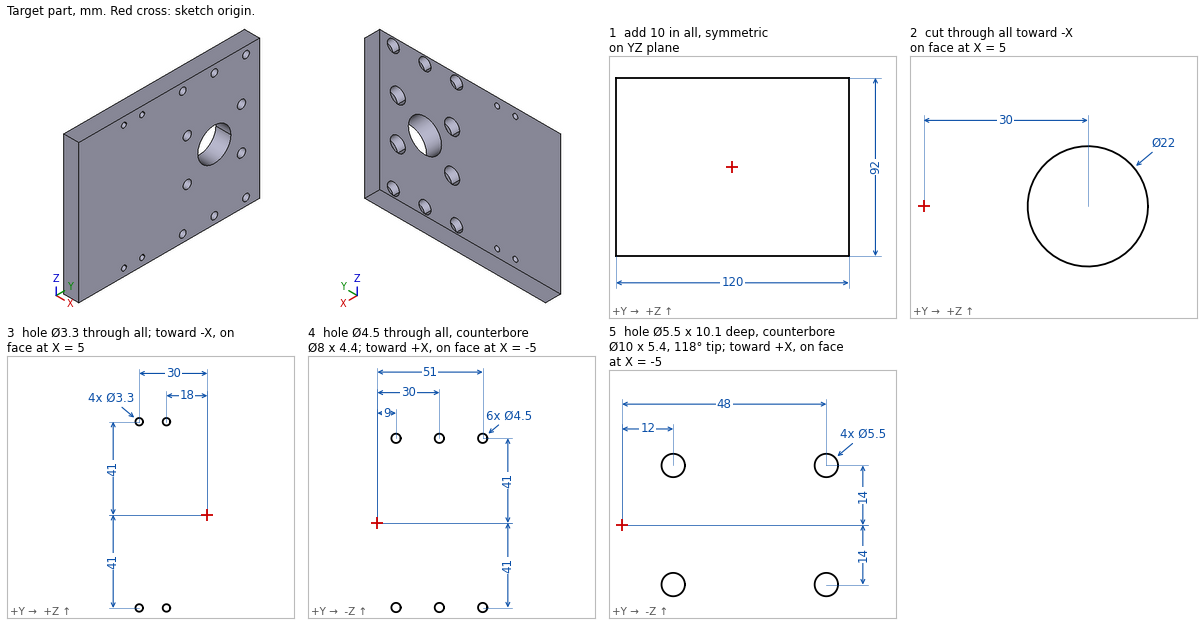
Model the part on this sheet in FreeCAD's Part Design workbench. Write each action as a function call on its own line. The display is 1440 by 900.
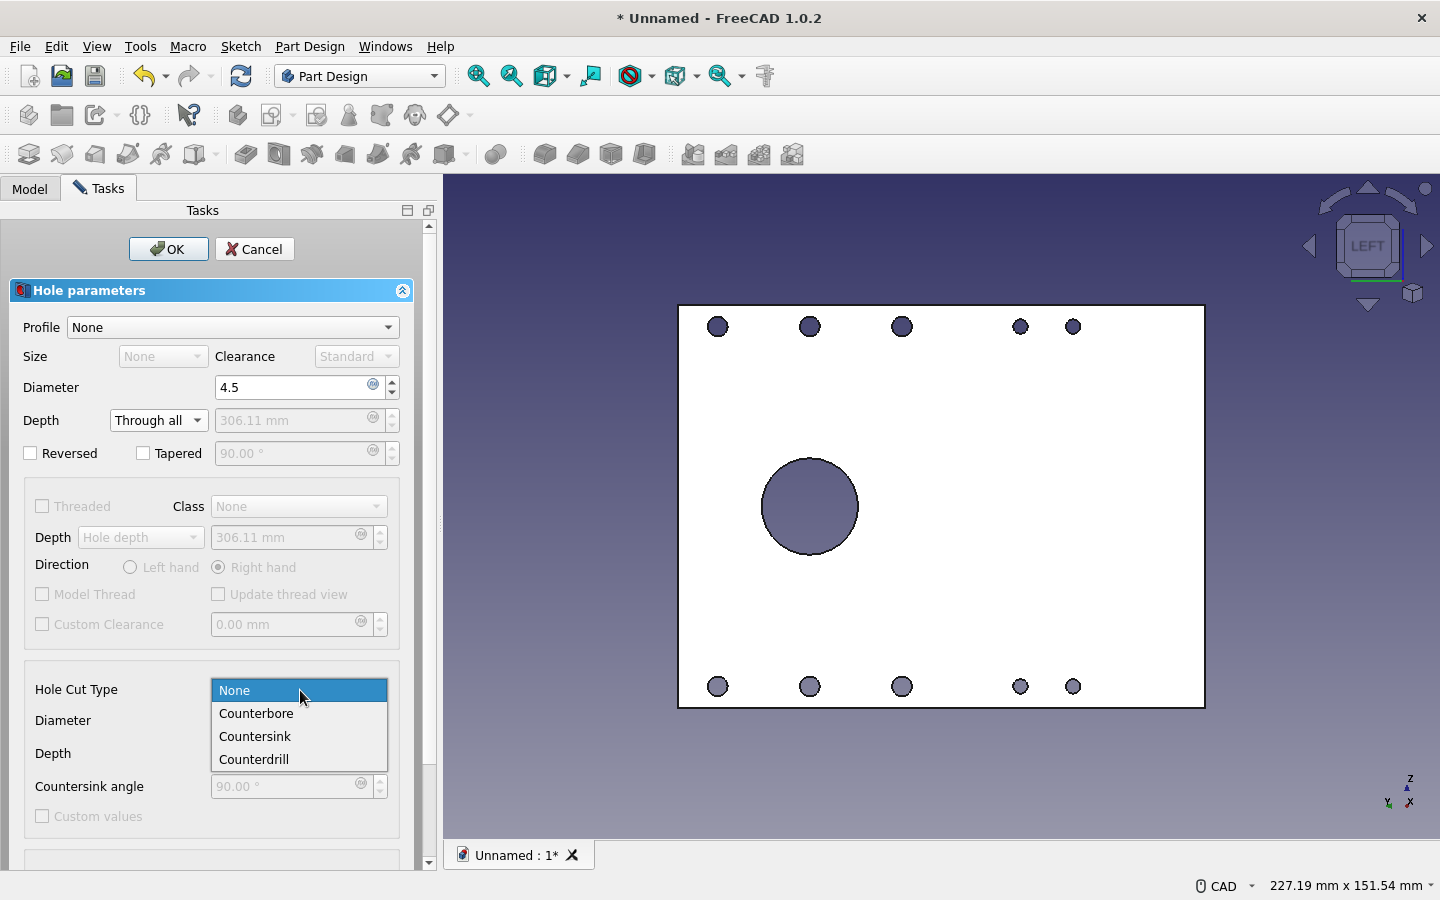
click(298, 714)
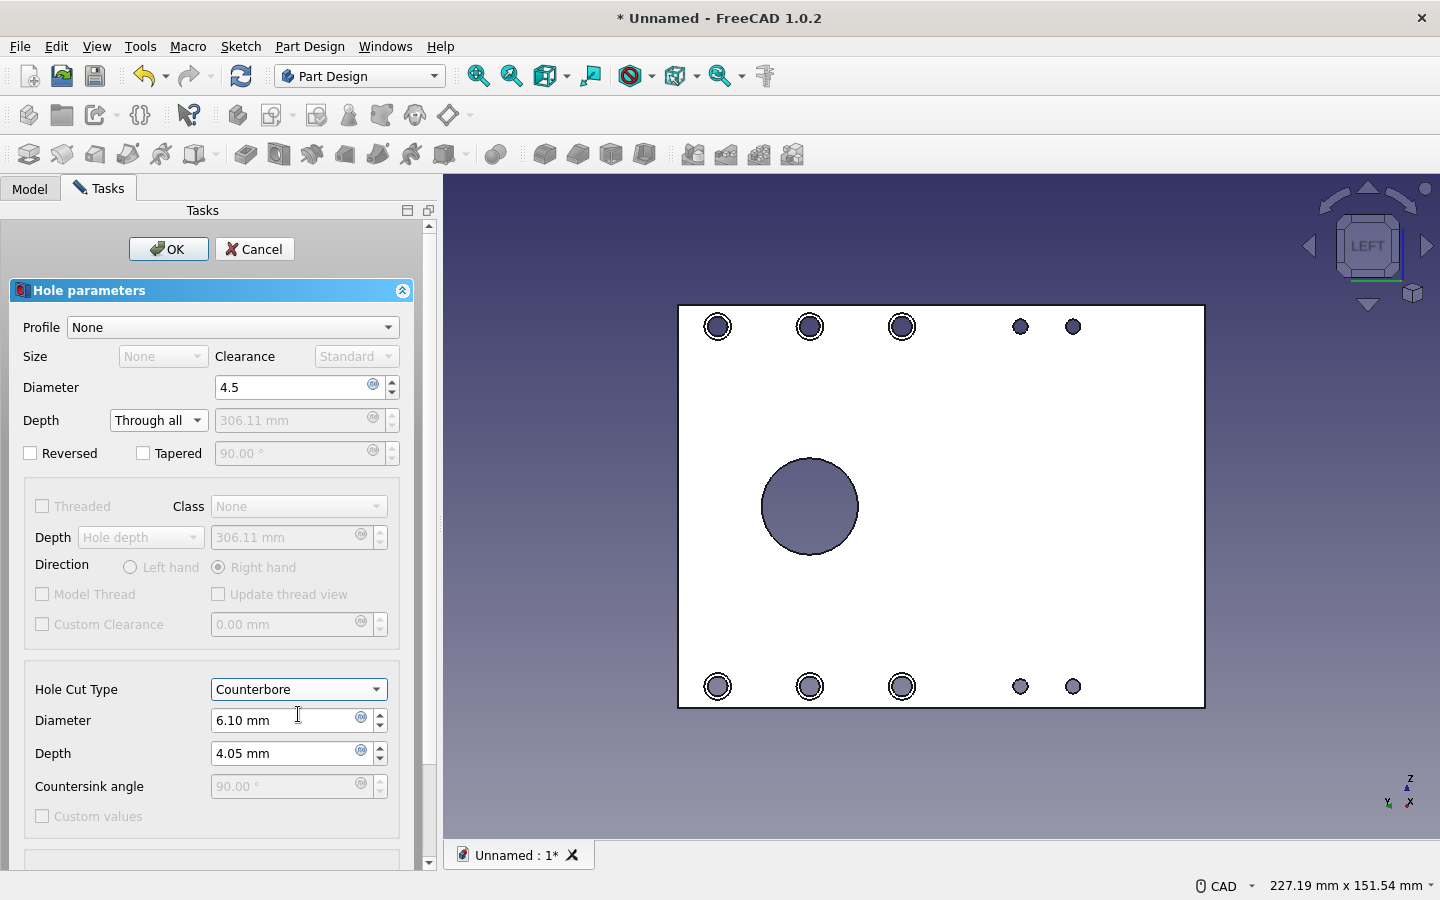
triple_click(292, 720)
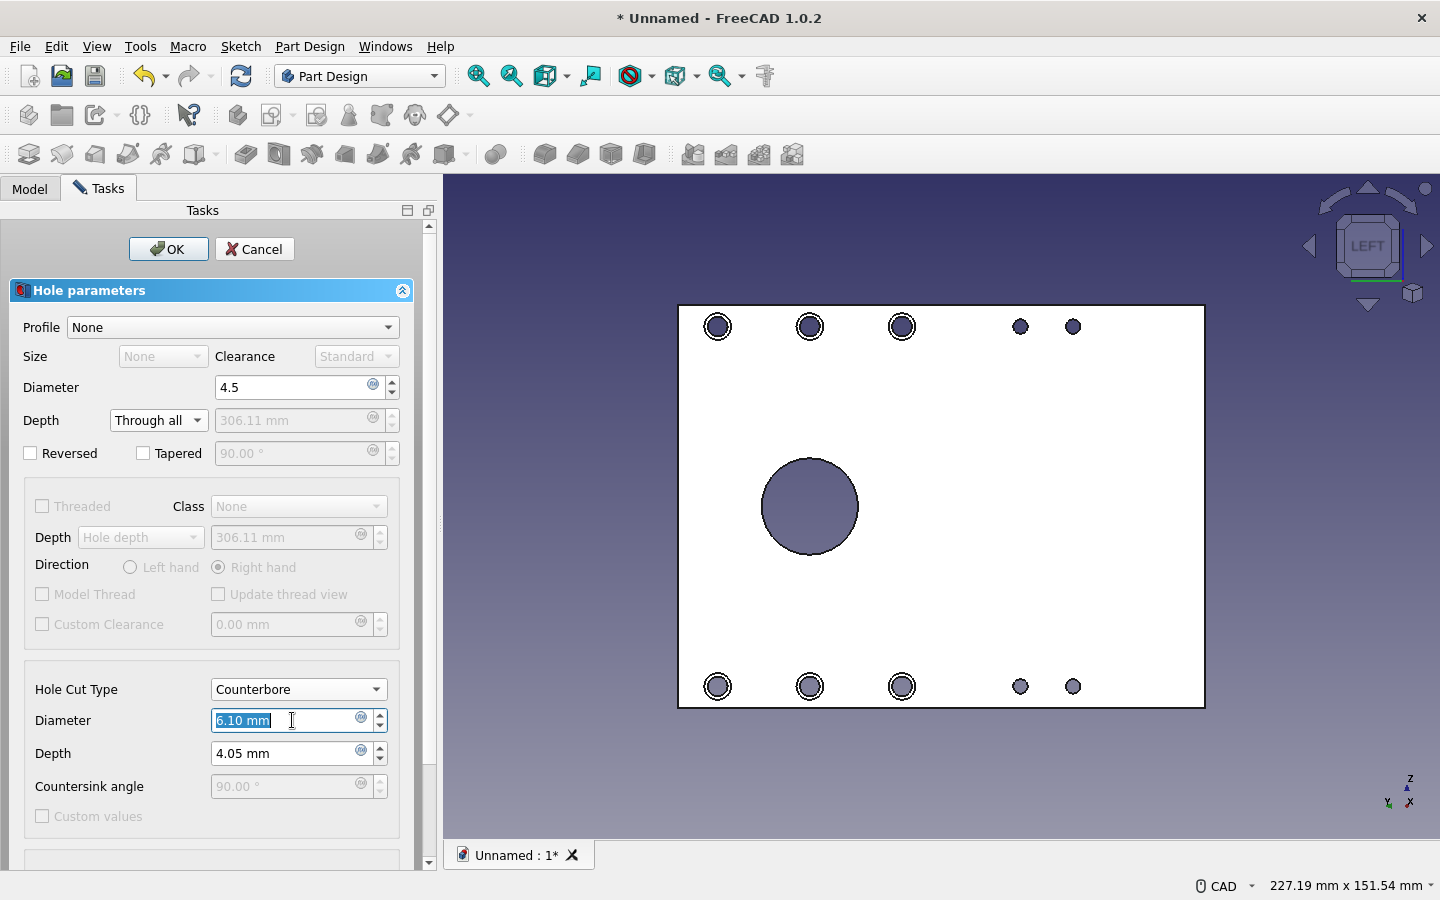
text(8)
key(Tab)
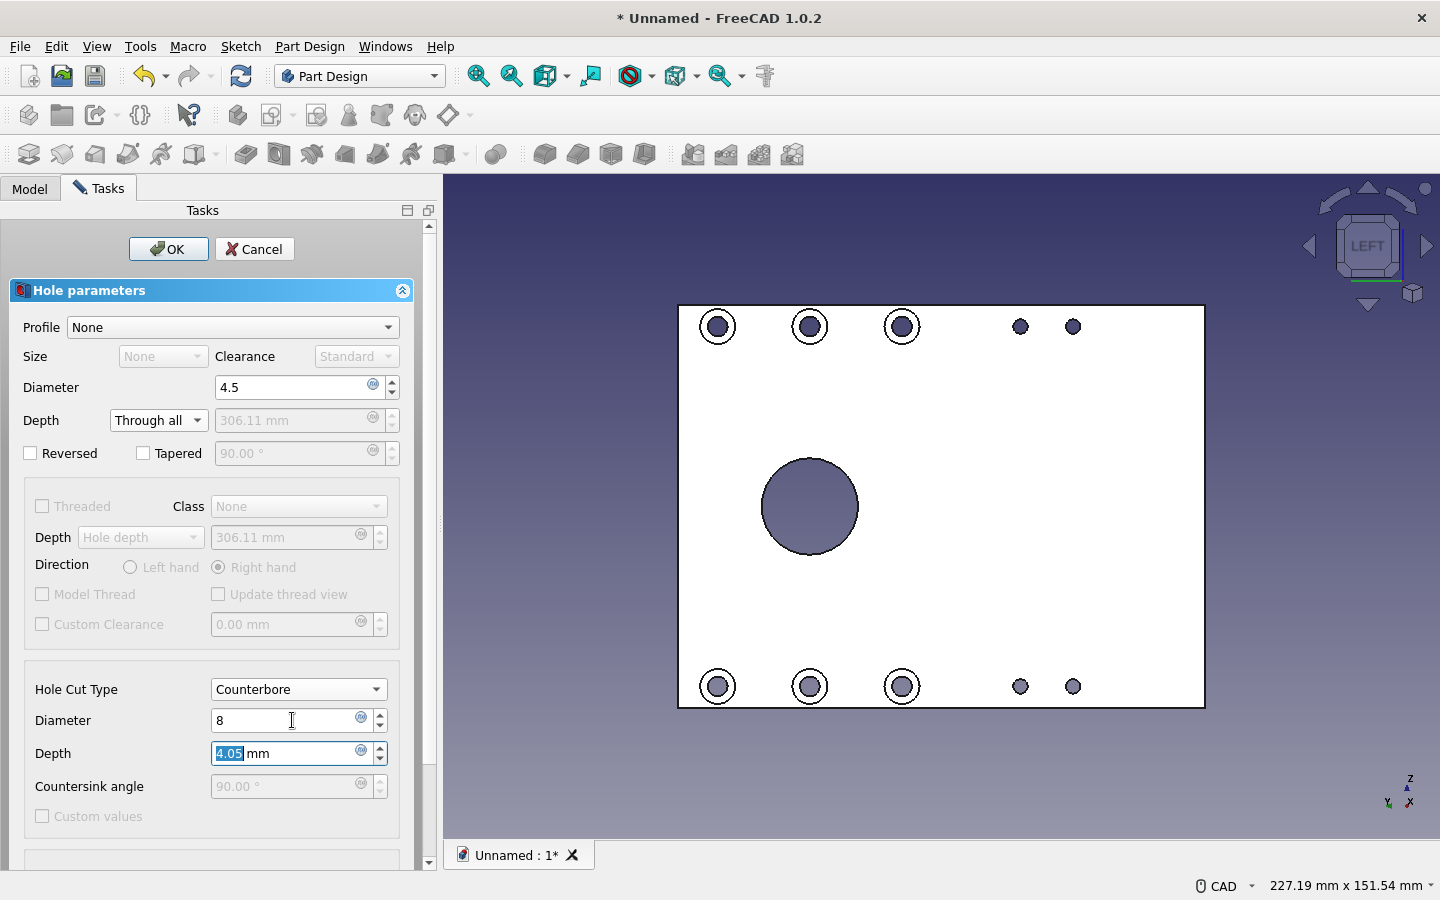
text(4.4)
key(Tab)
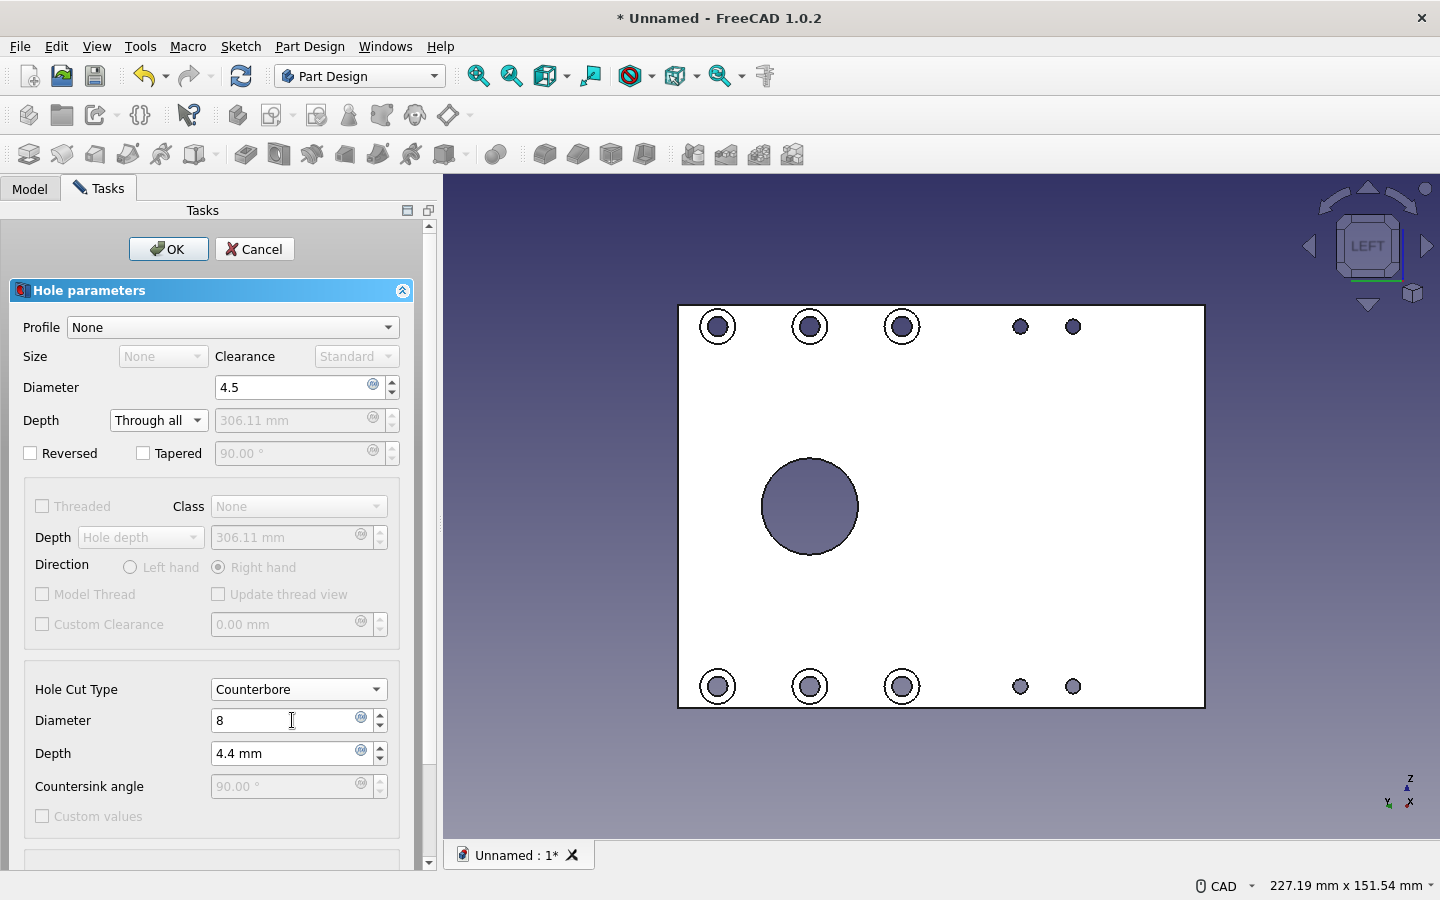
click(169, 249)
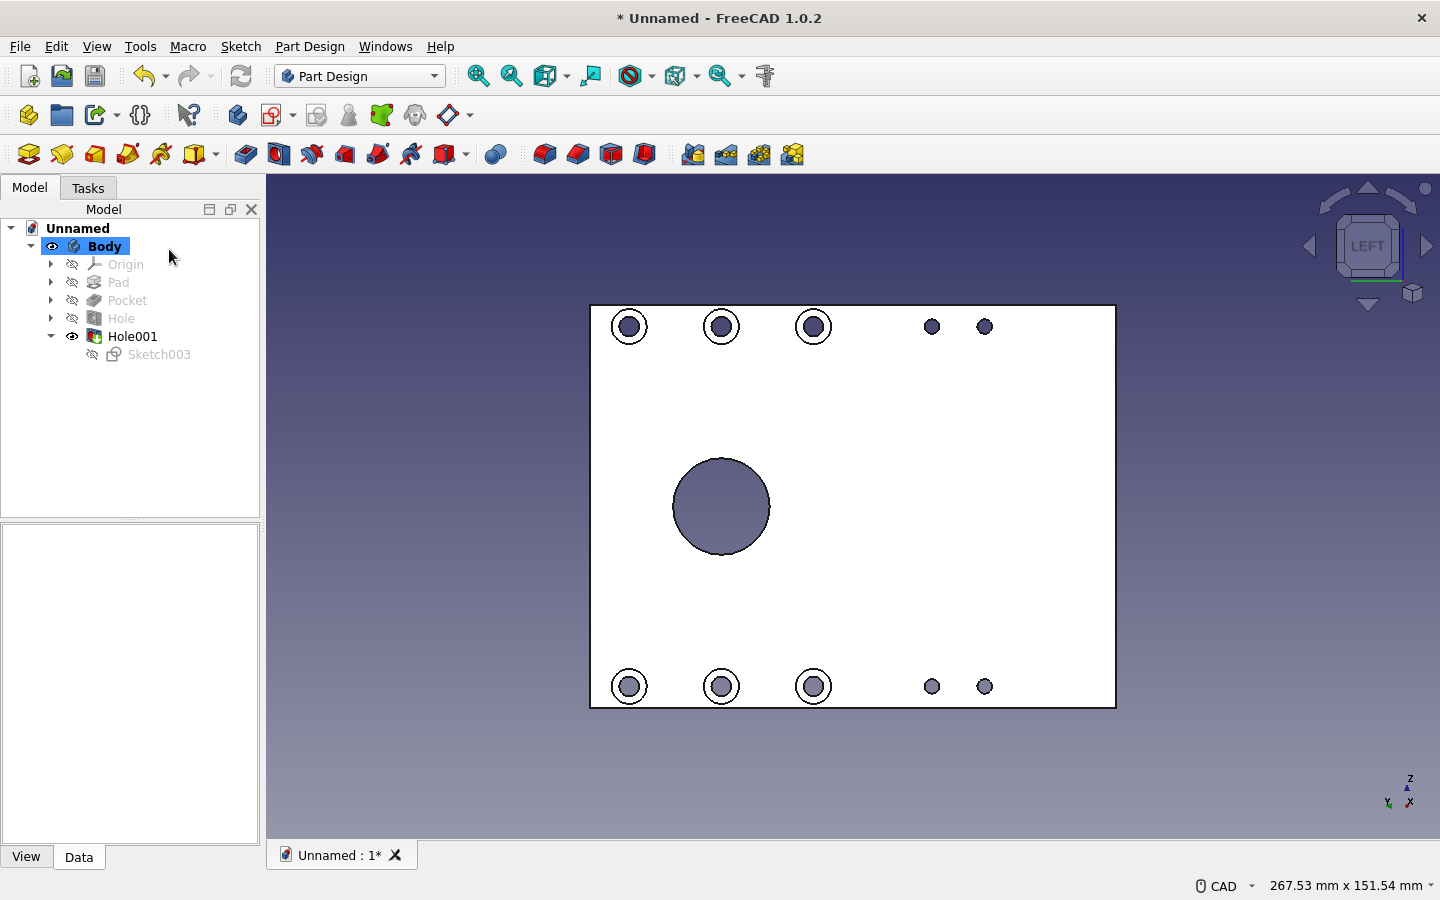
click(928, 505)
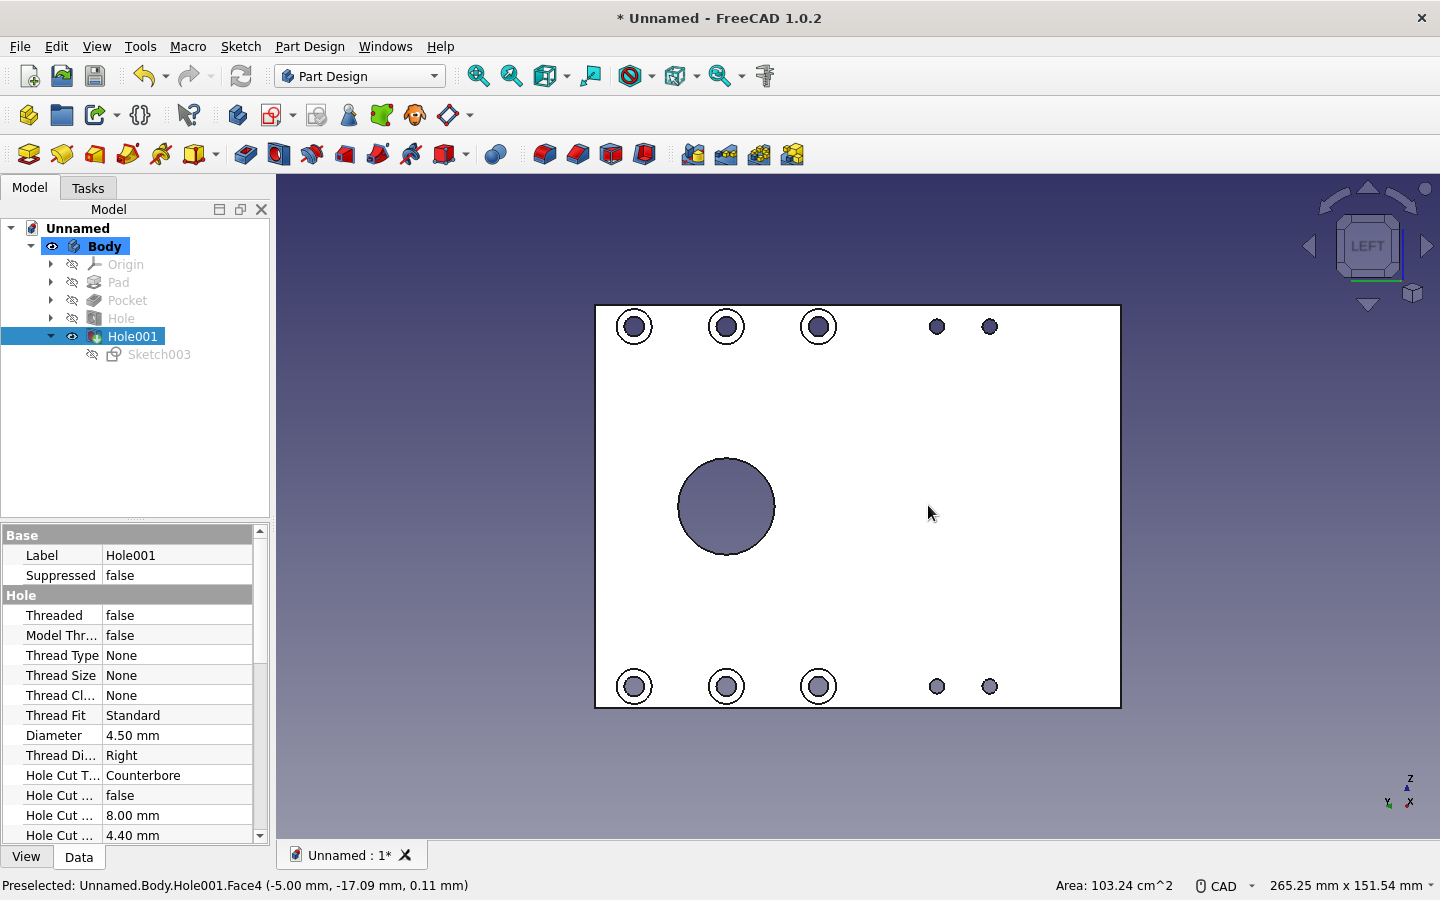
click(270, 116)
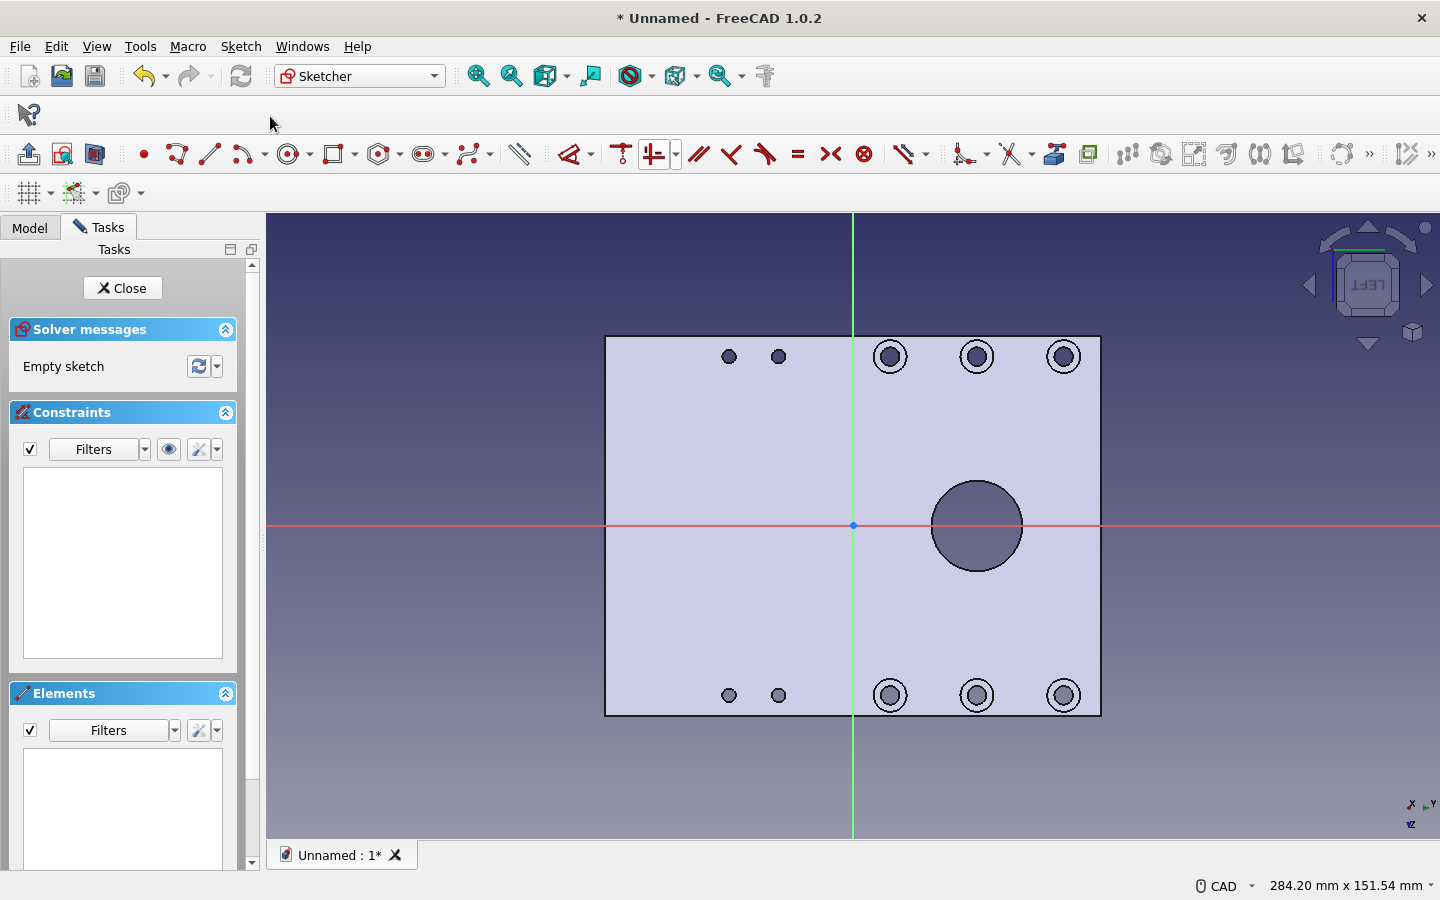
scroll(1059, 526, up, 5)